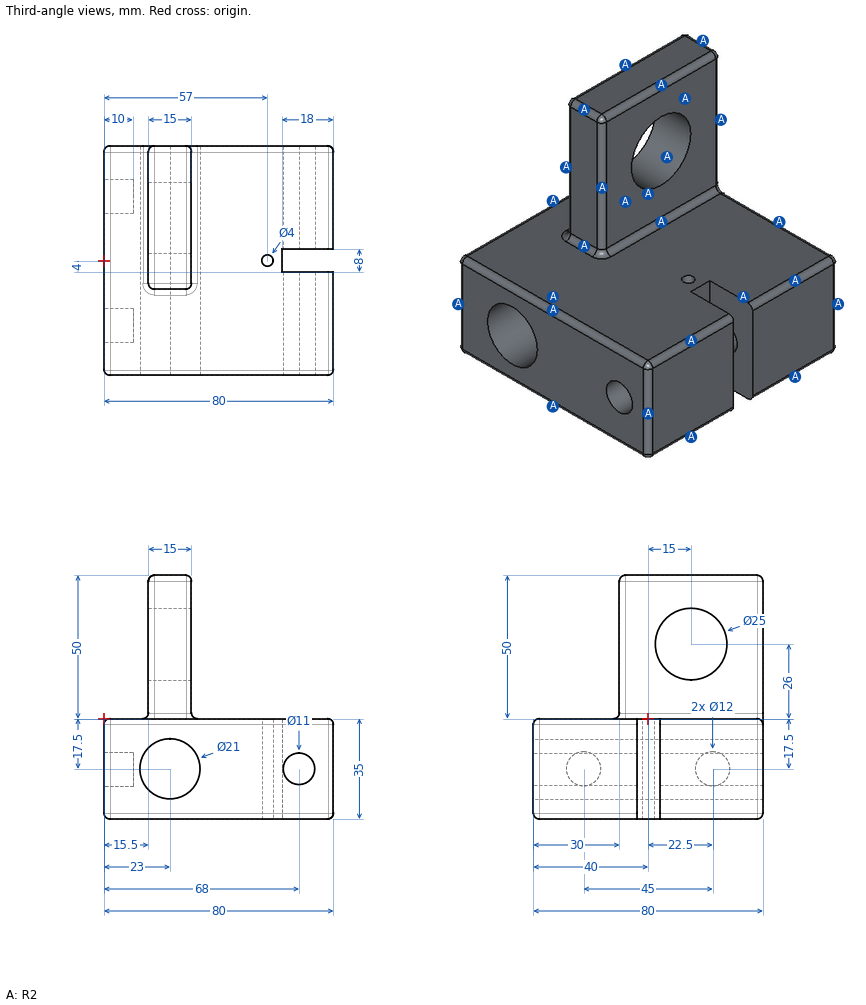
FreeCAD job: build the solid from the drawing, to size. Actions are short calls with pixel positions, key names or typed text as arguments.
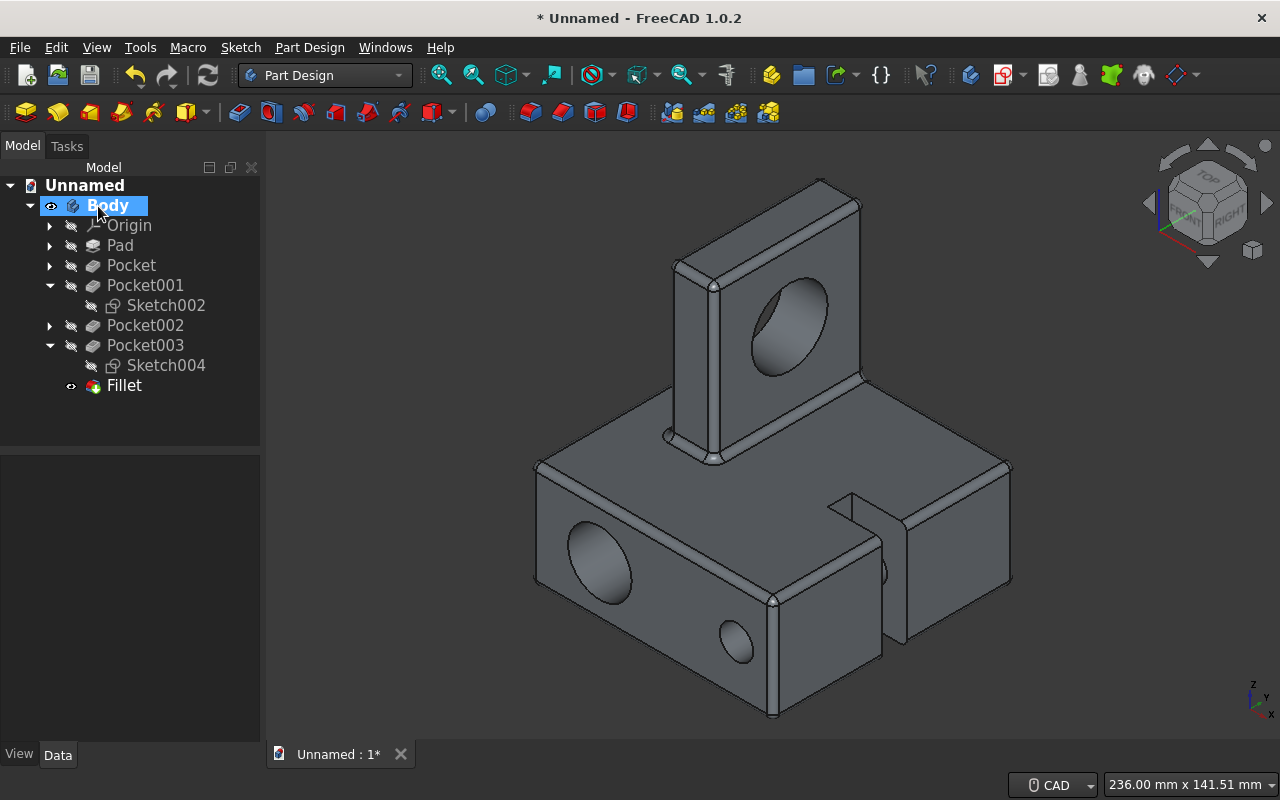
click(1004, 76)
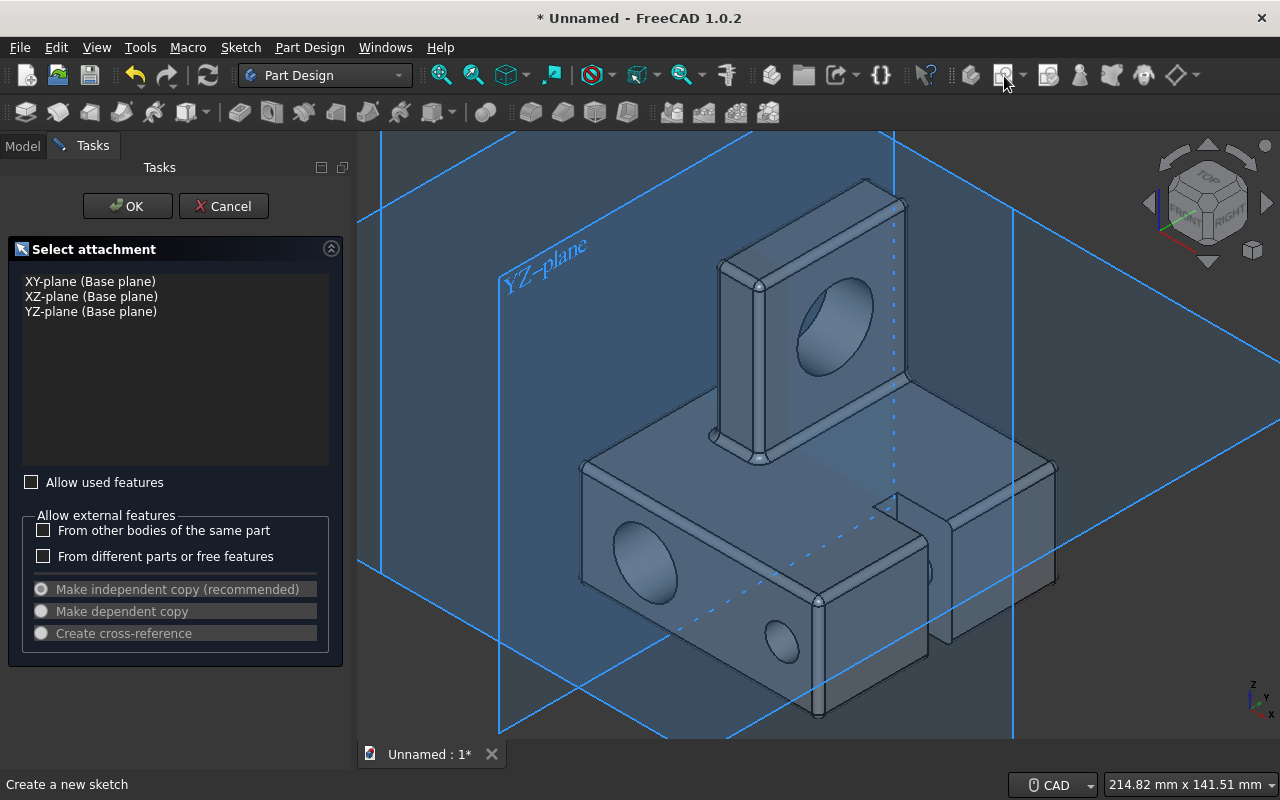
click(82, 282)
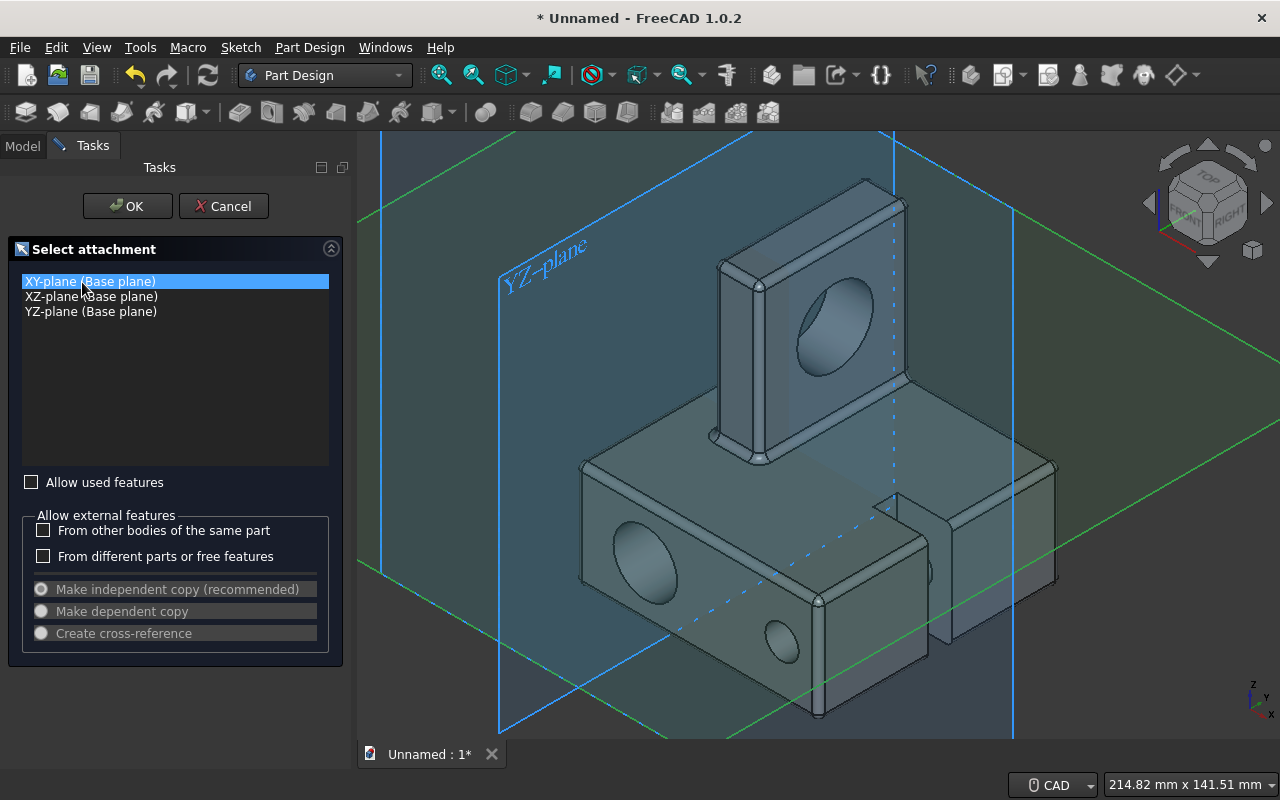
click(128, 206)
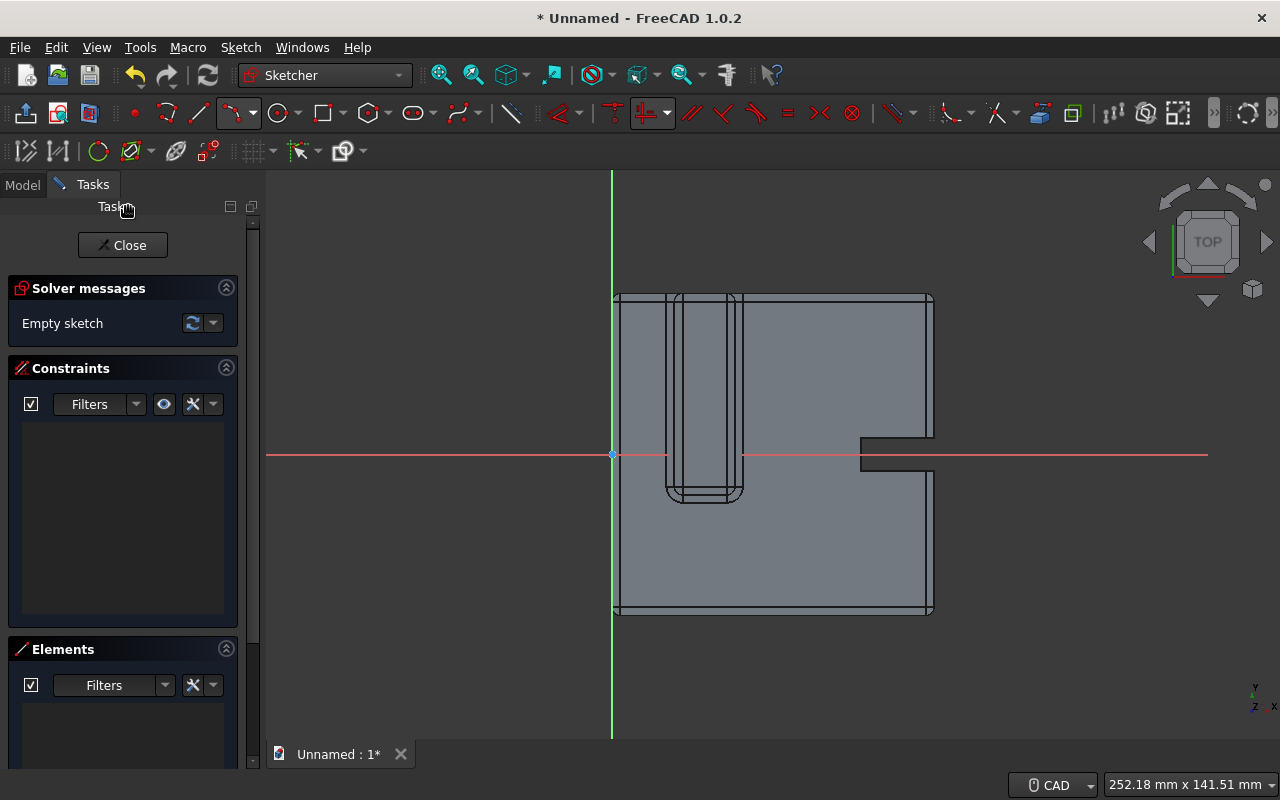
click(90, 114)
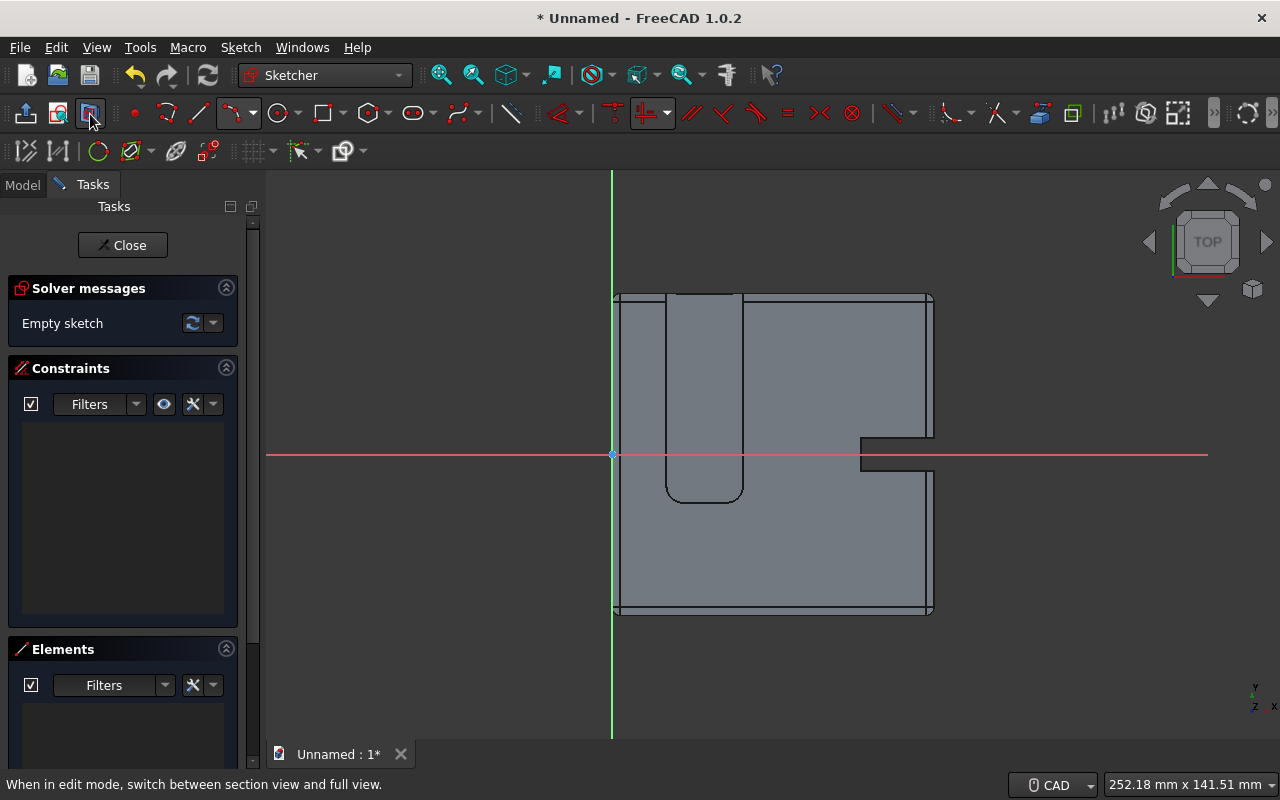
scroll(849, 455, up, 15)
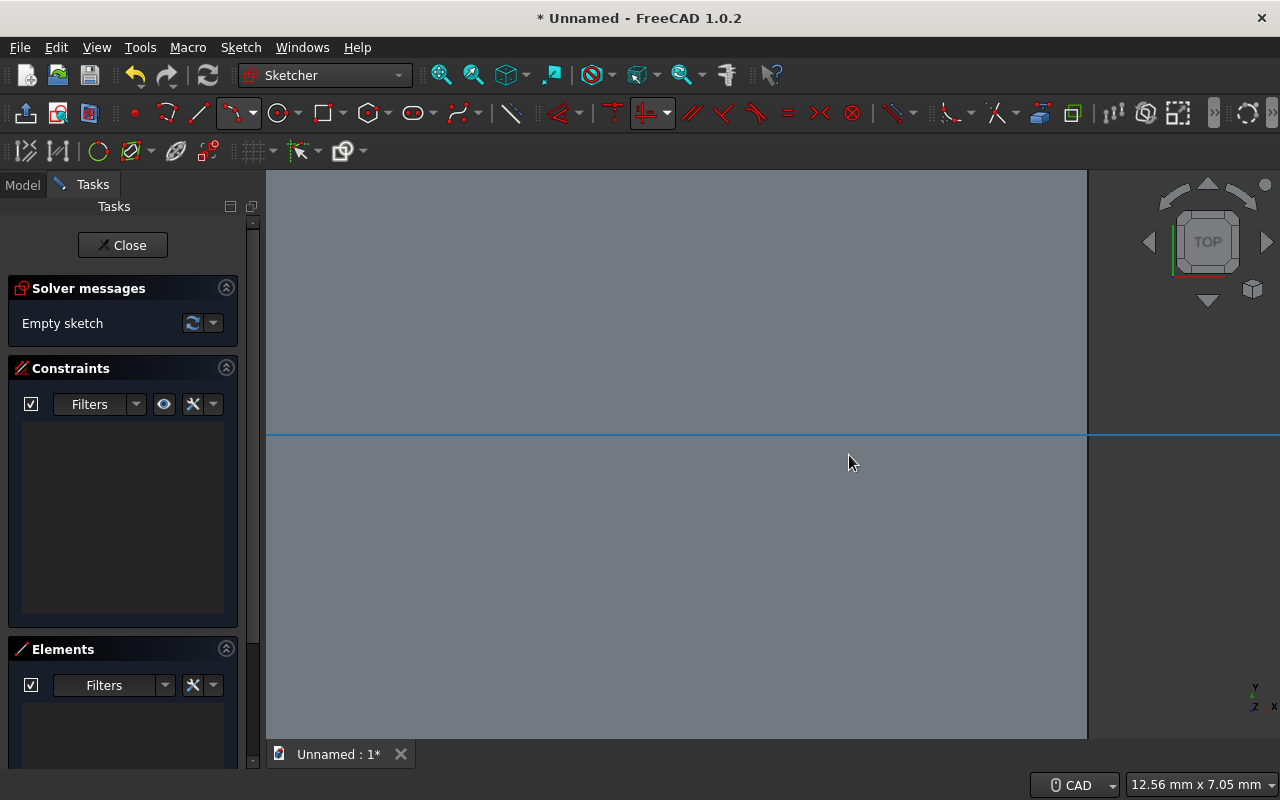
click(278, 114)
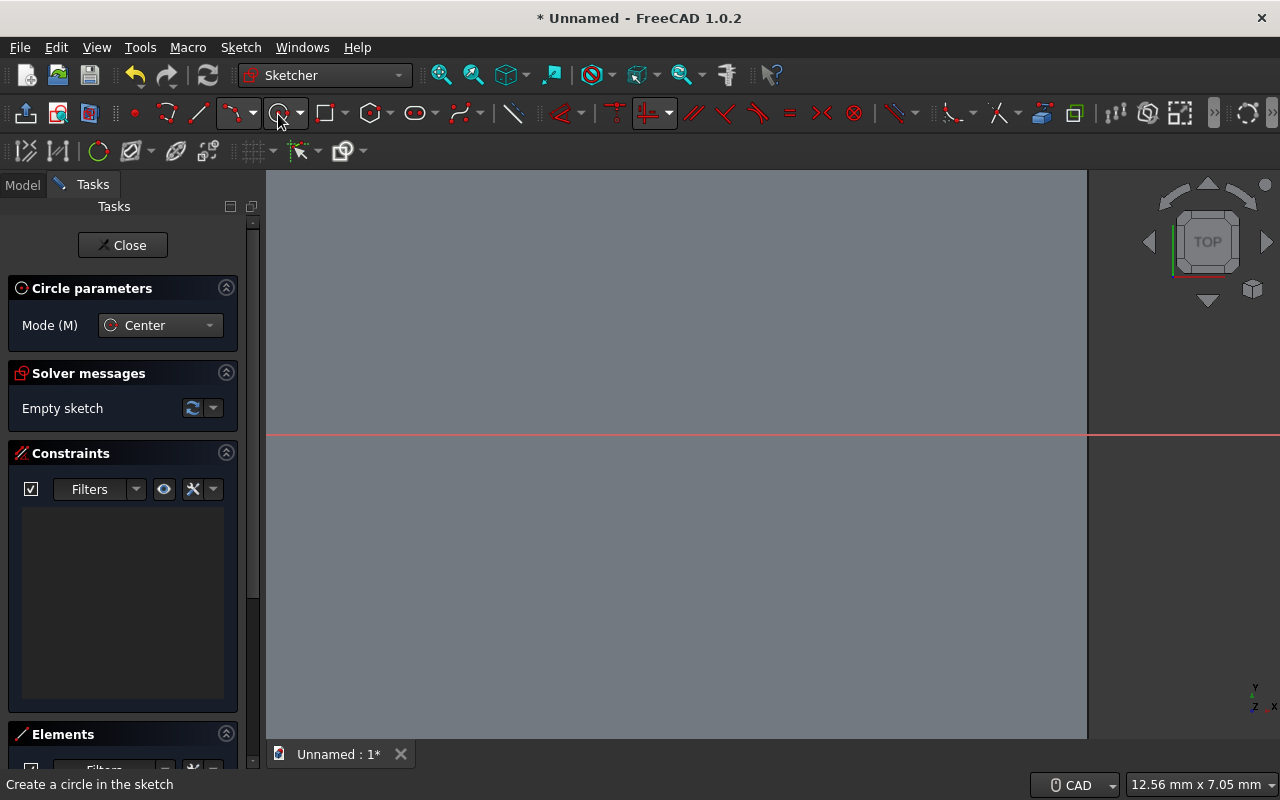
click(684, 435)
click(799, 321)
key(Escape)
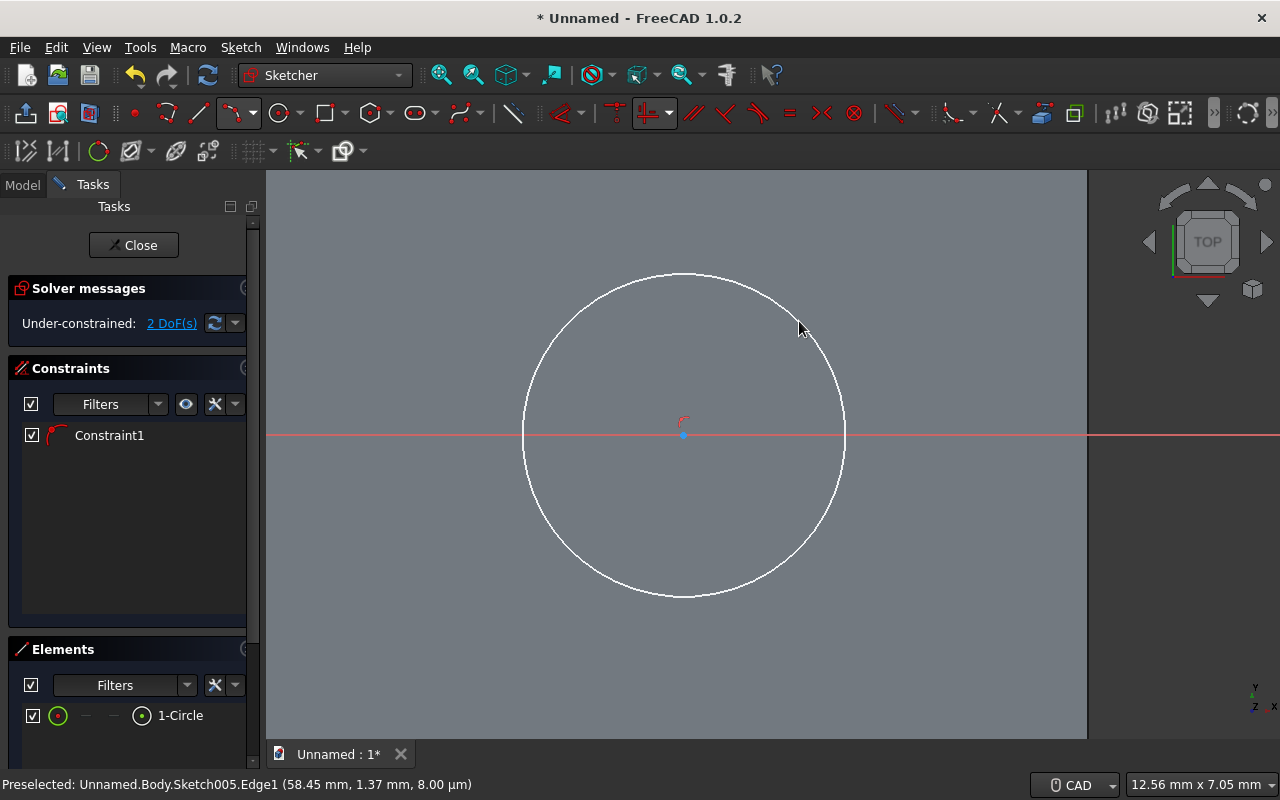
click(560, 114)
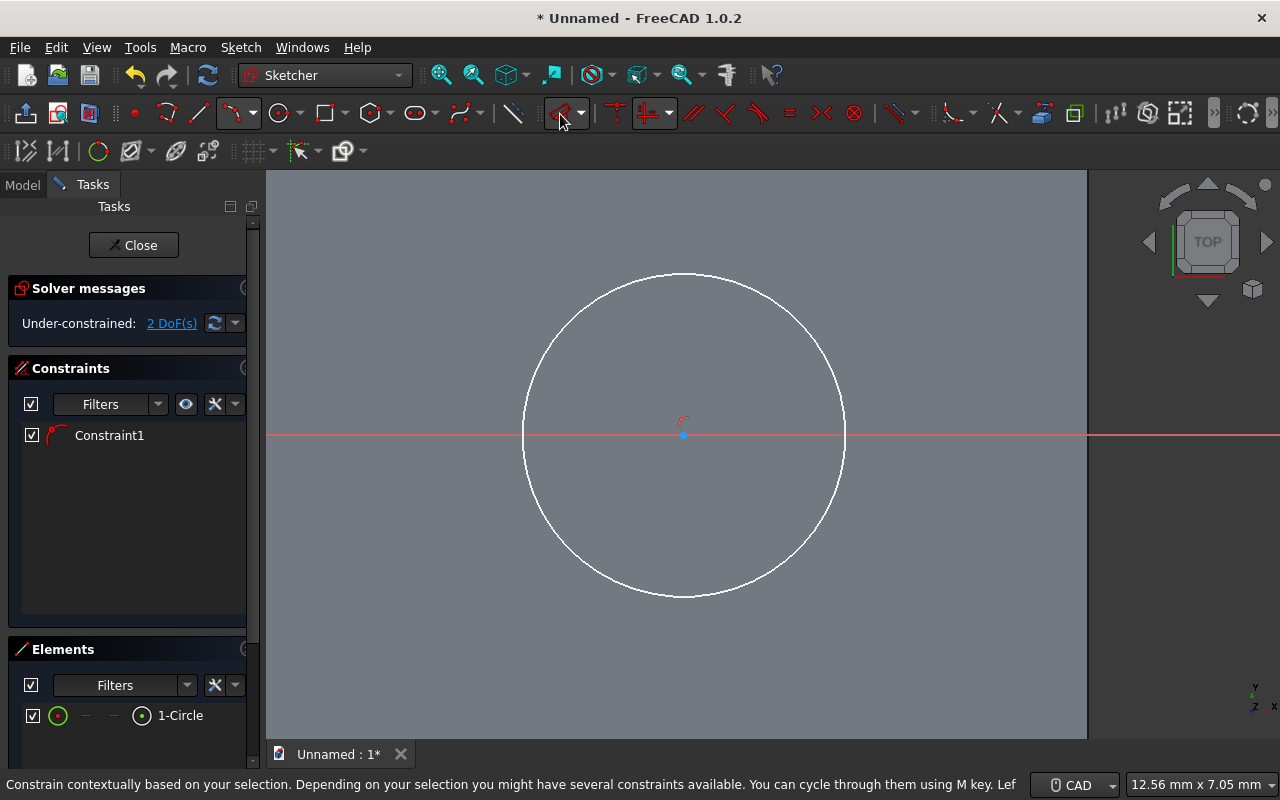
click(798, 321)
click(821, 298)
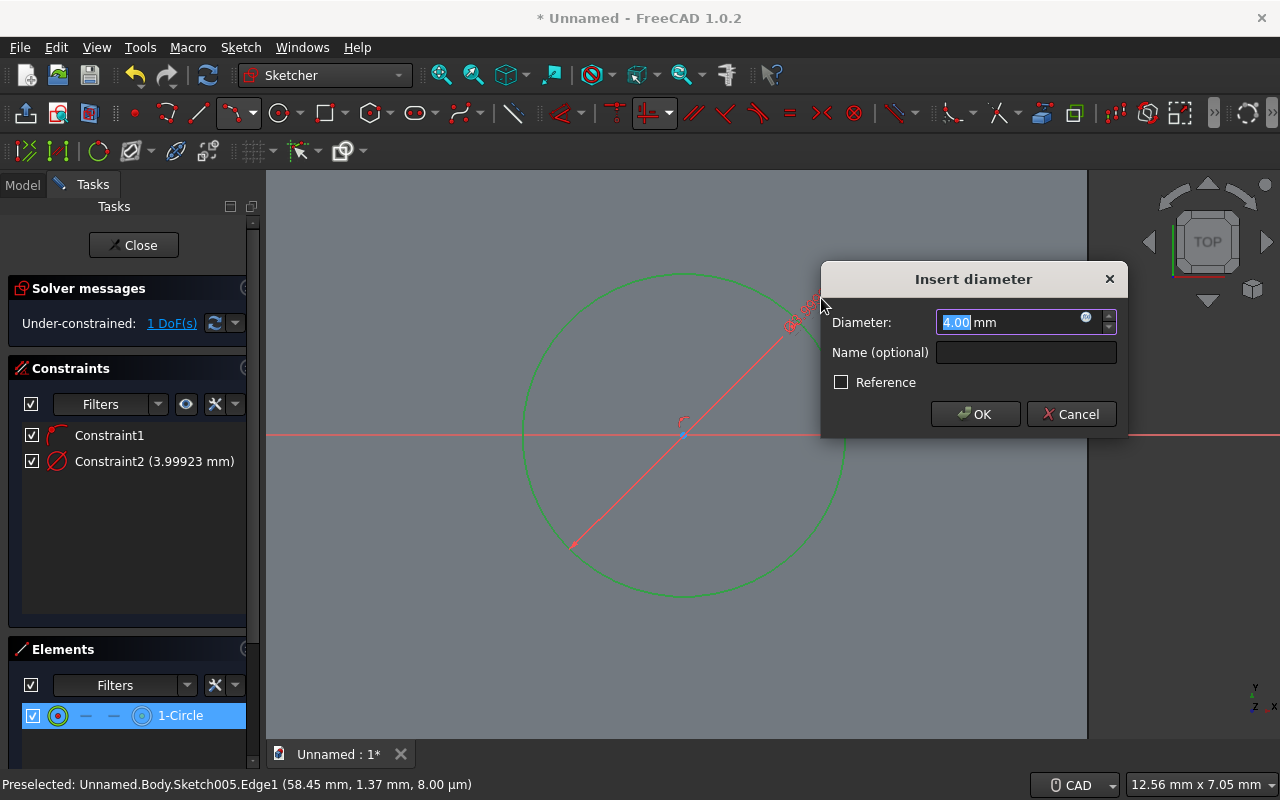
text(4)
key(Return)